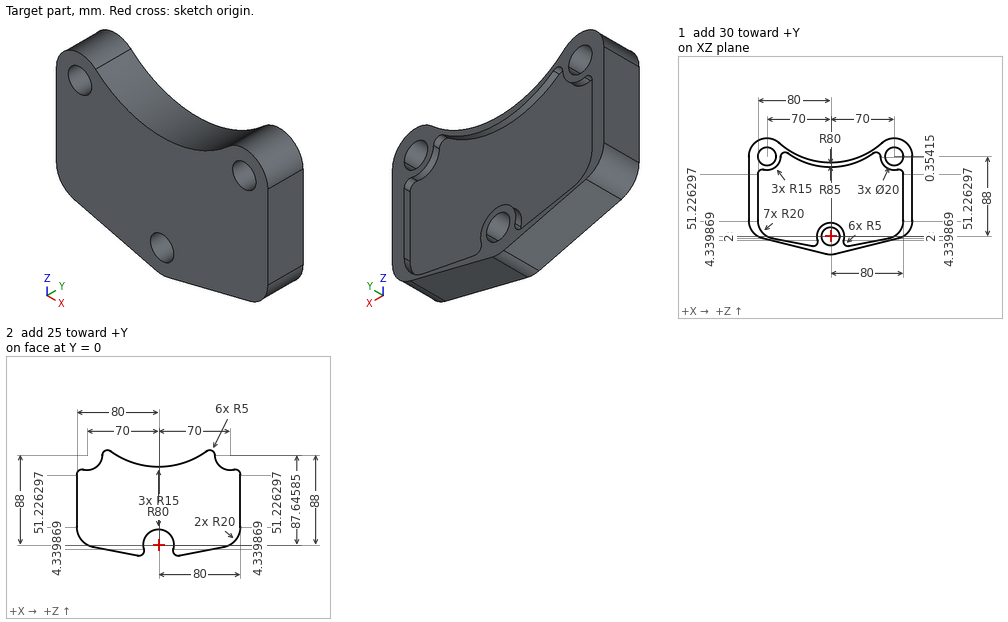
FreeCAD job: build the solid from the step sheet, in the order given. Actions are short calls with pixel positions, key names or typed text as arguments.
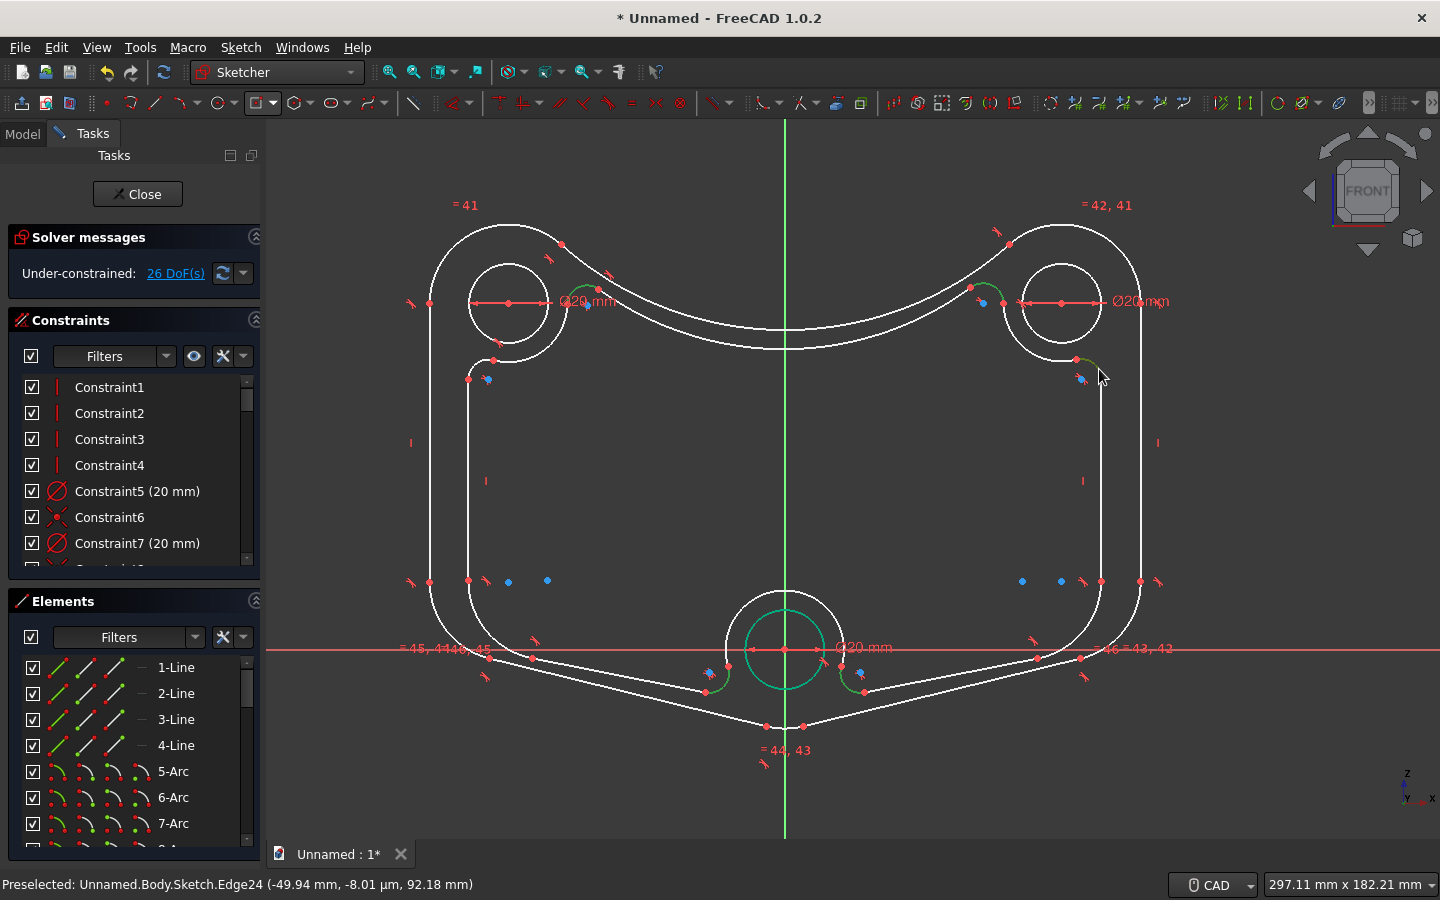
scroll(483, 360, up, 2)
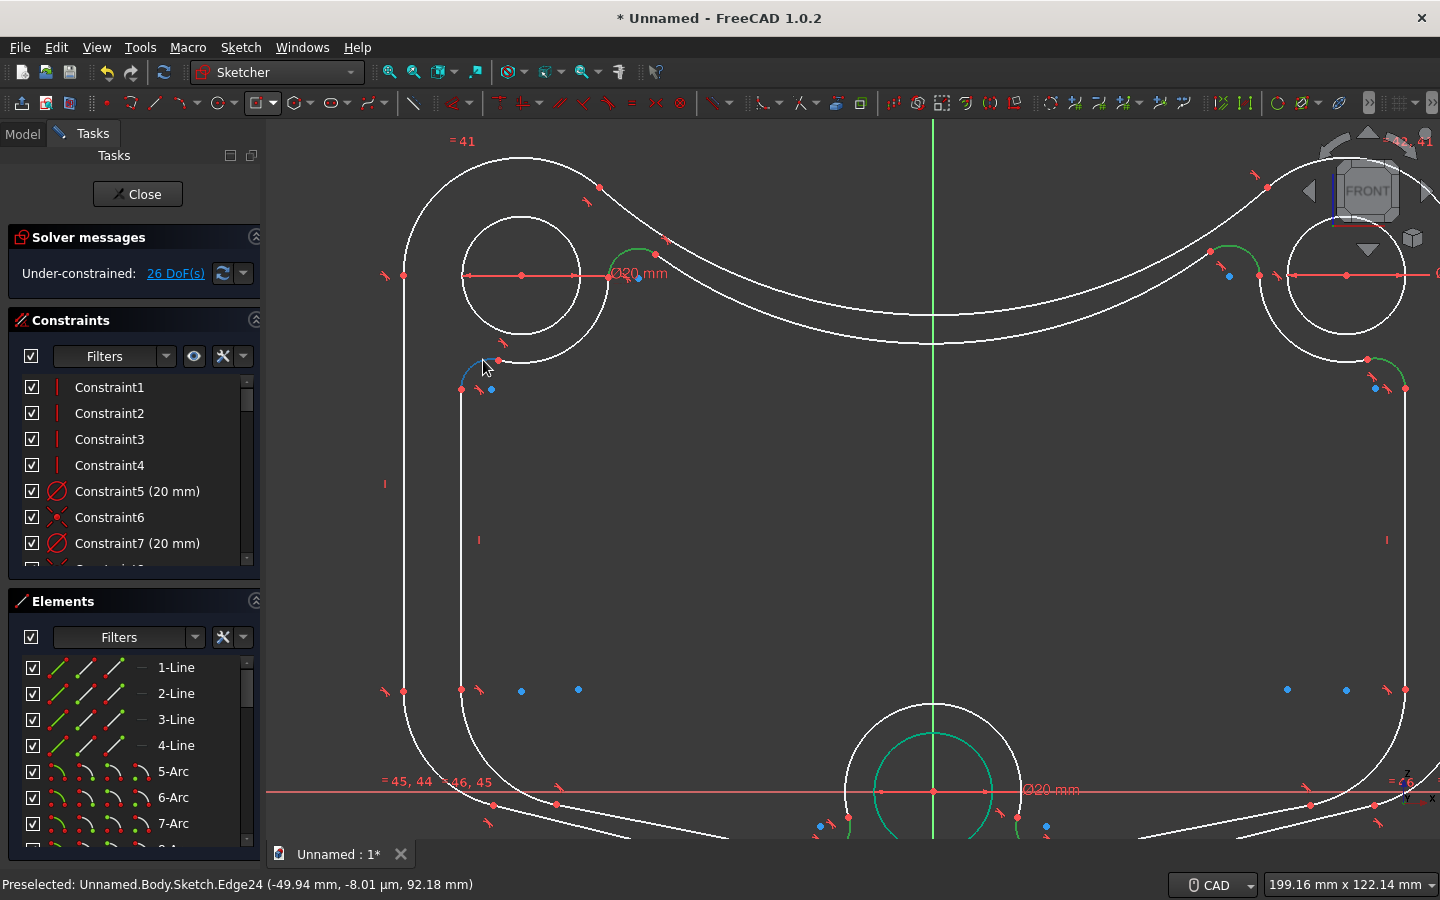
click(483, 360)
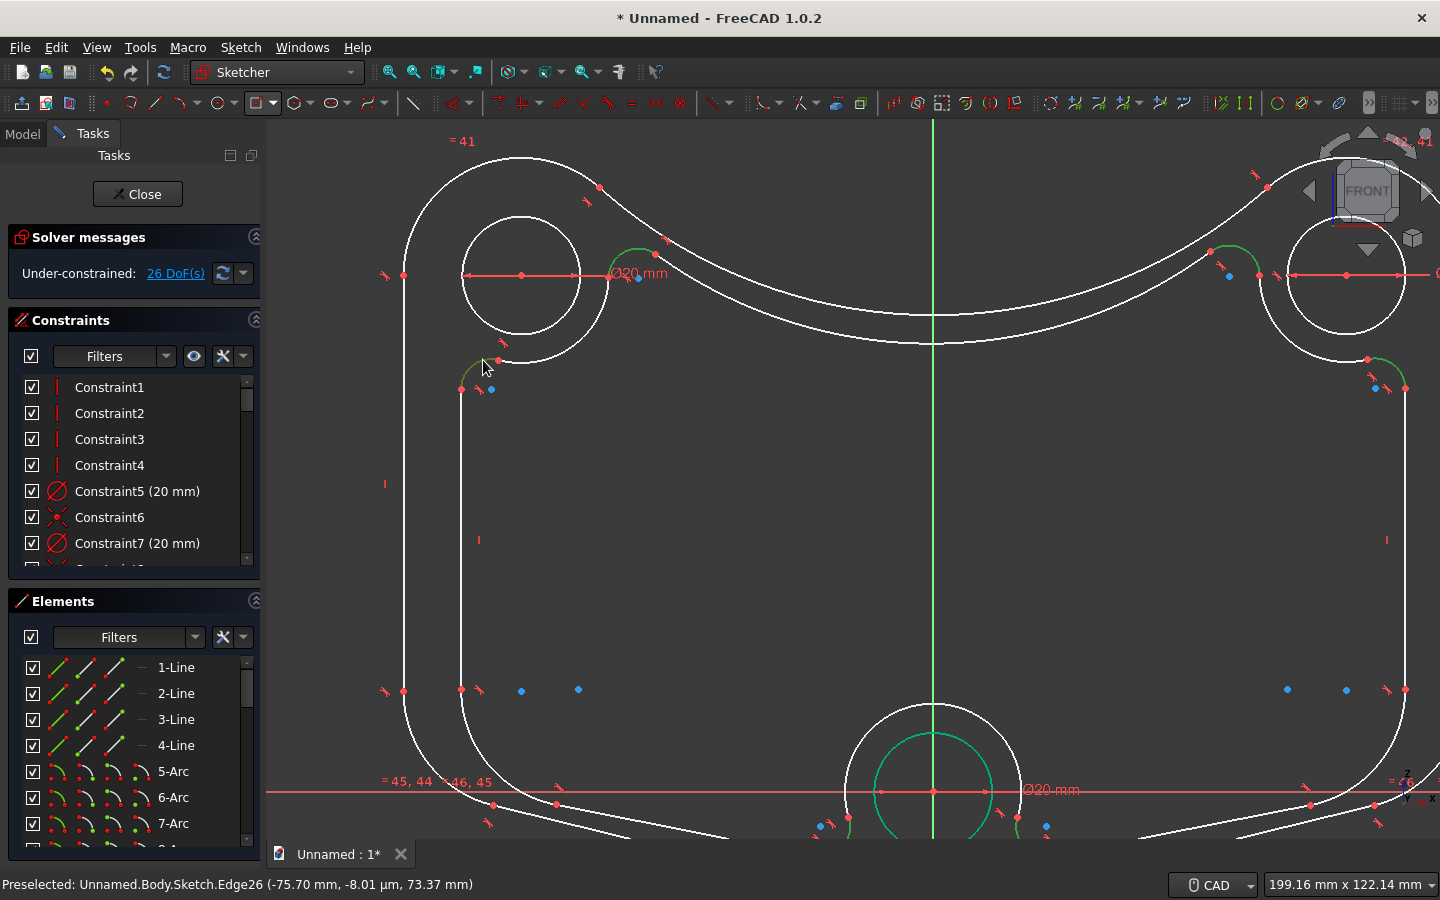
key(e)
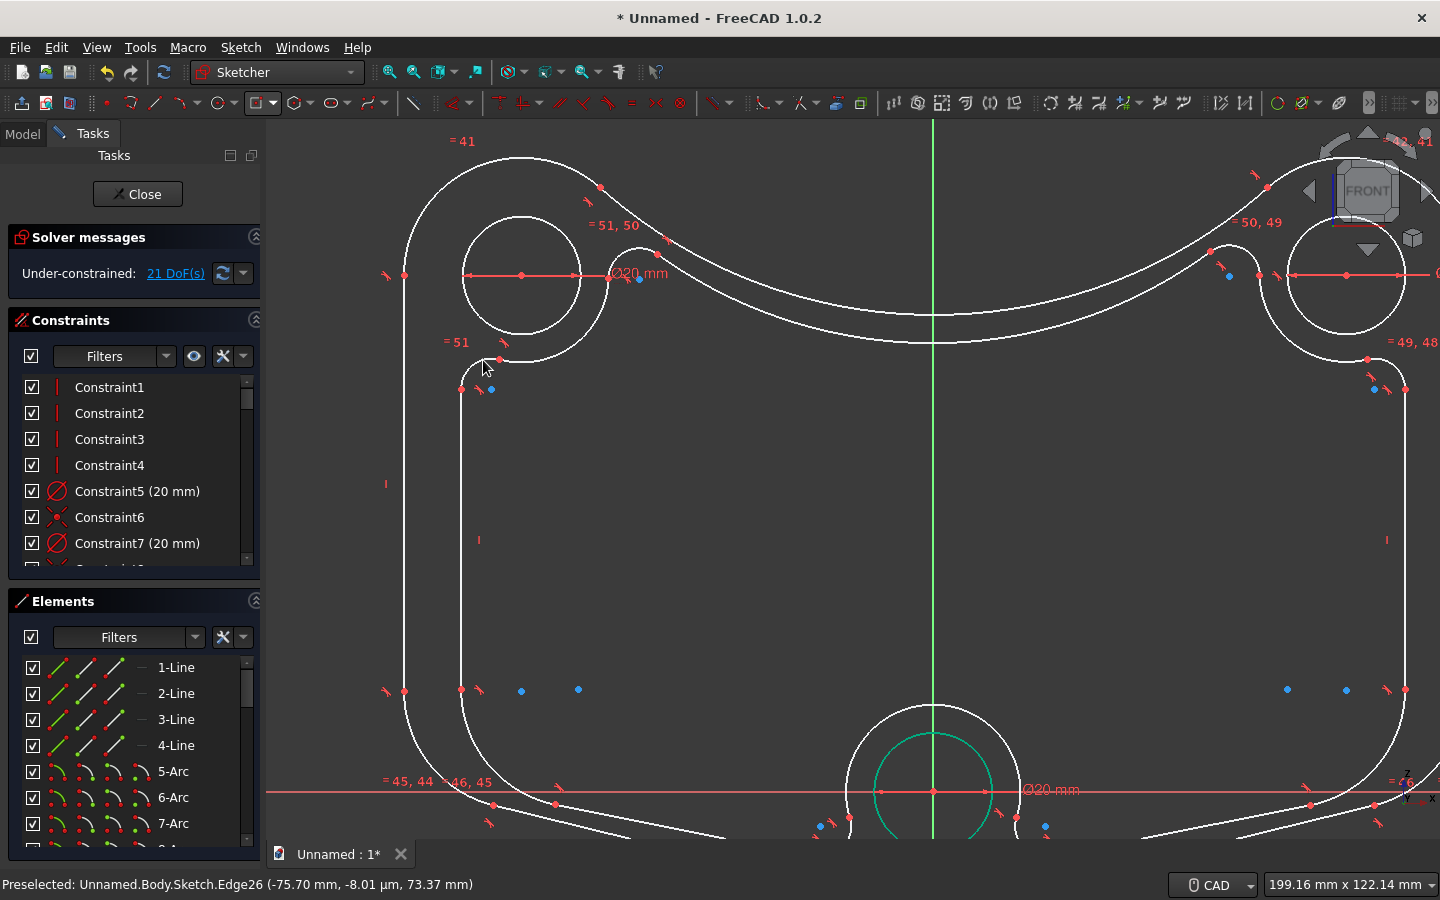
click(993, 728)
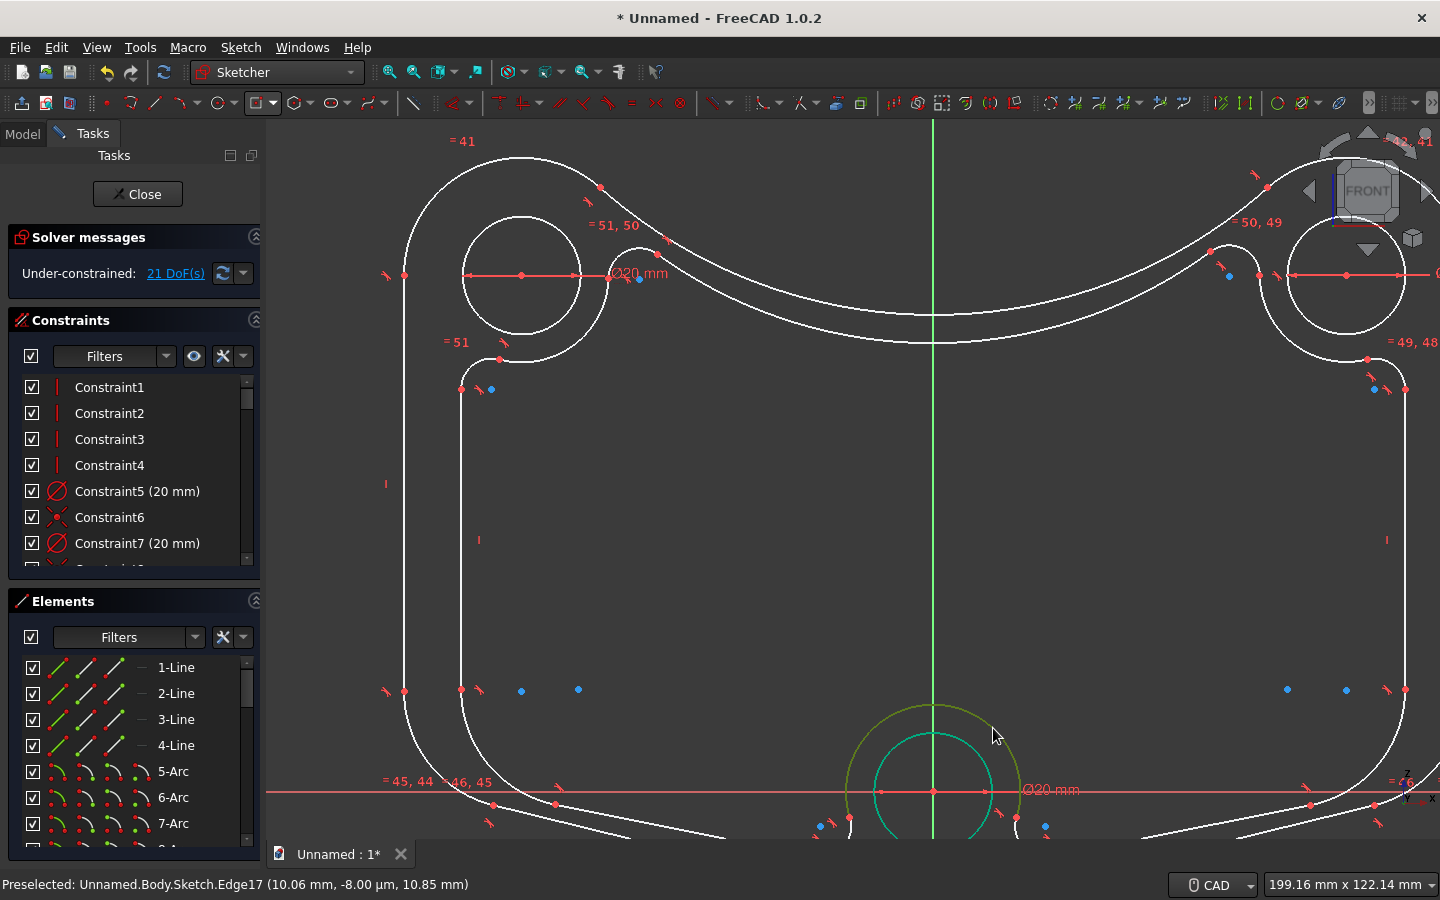
click(1272, 320)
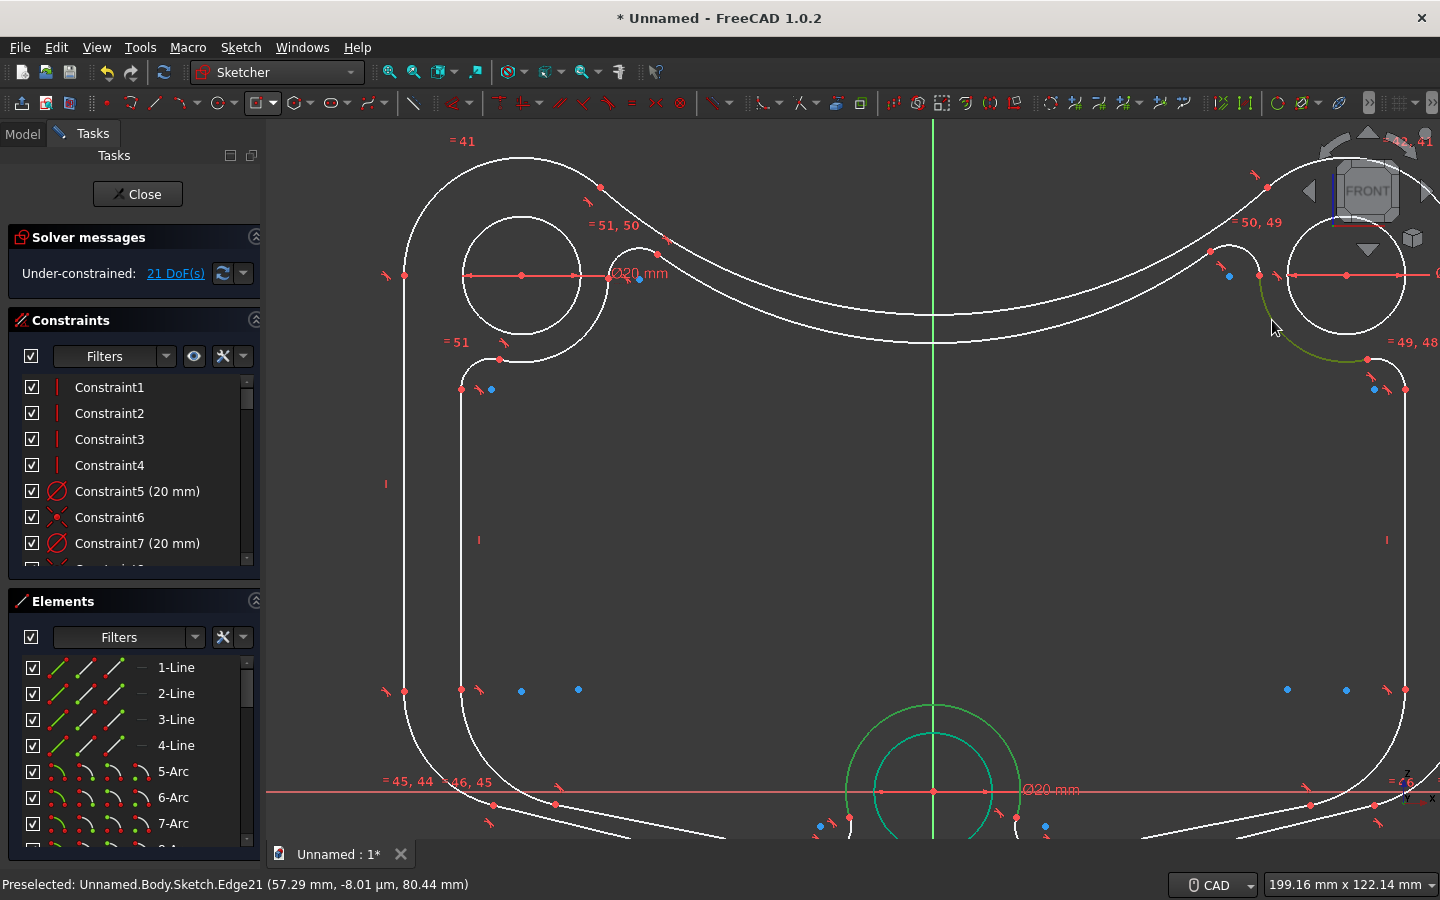
click(546, 359)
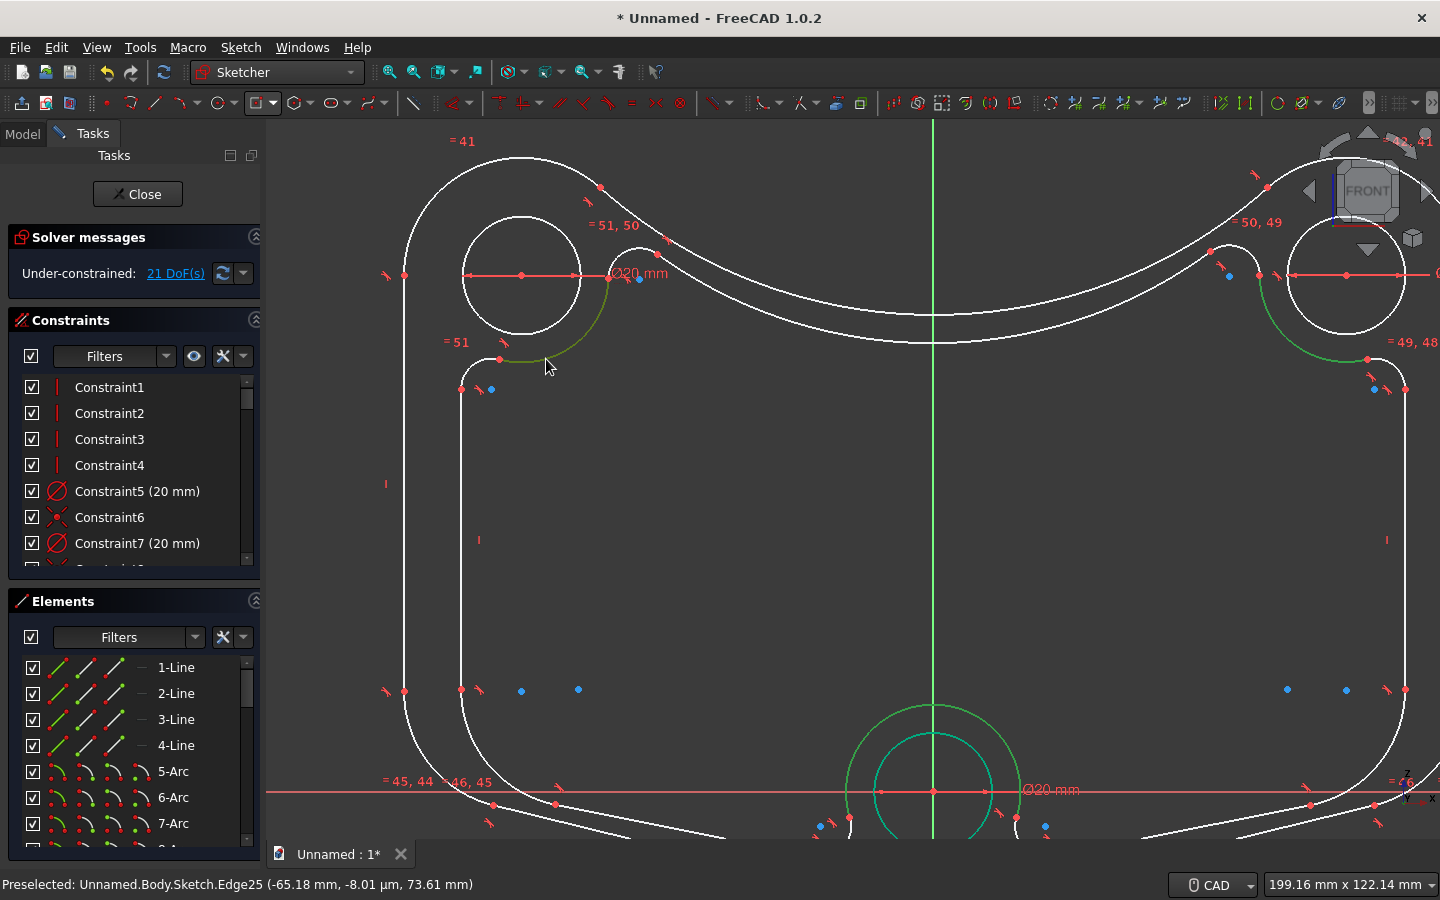
click(632, 104)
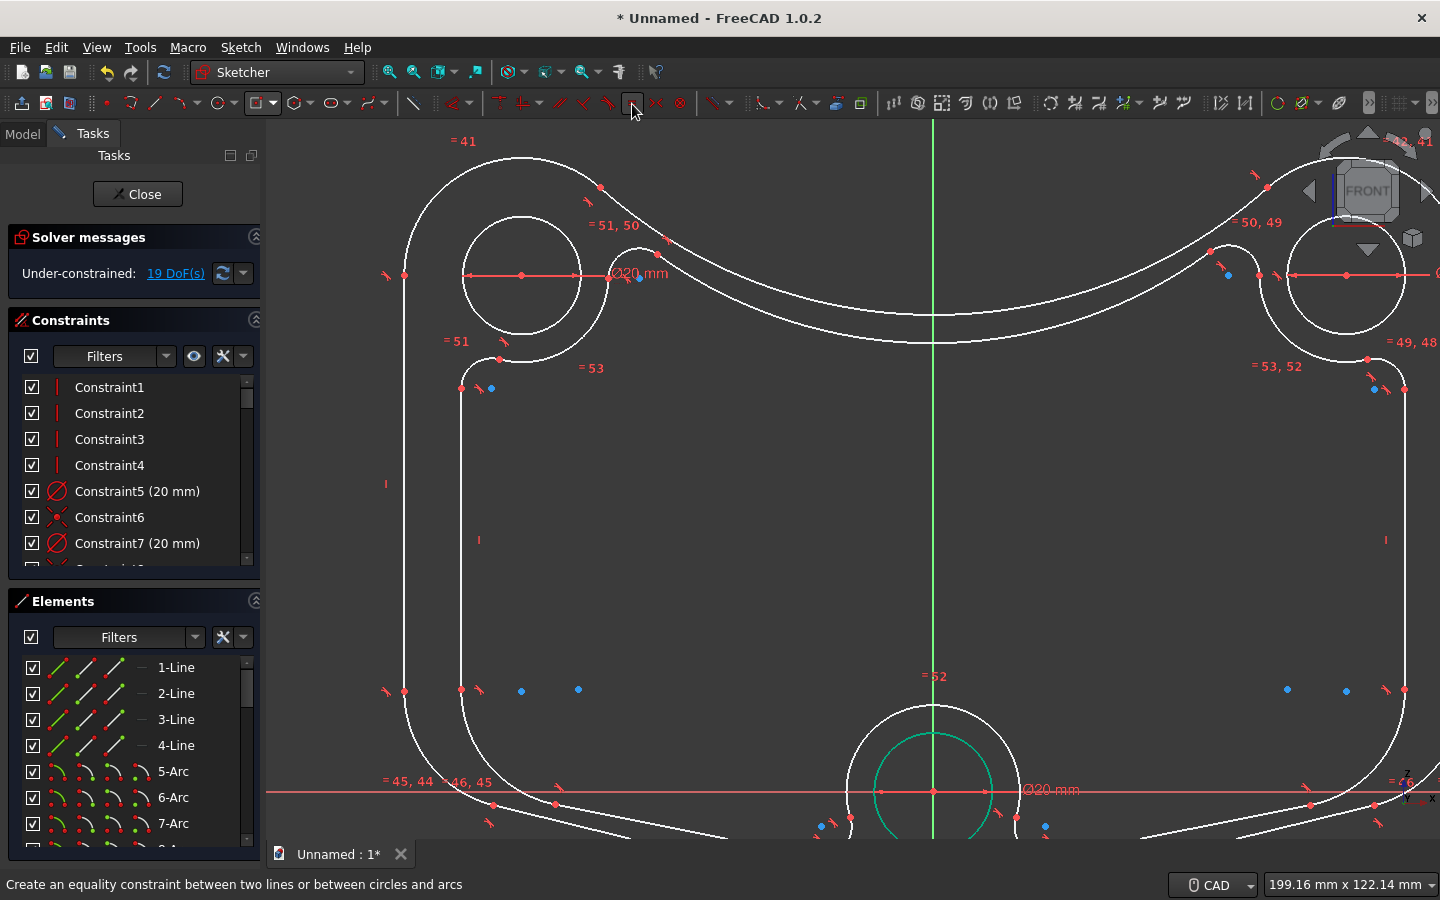
scroll(482, 360, down, 2)